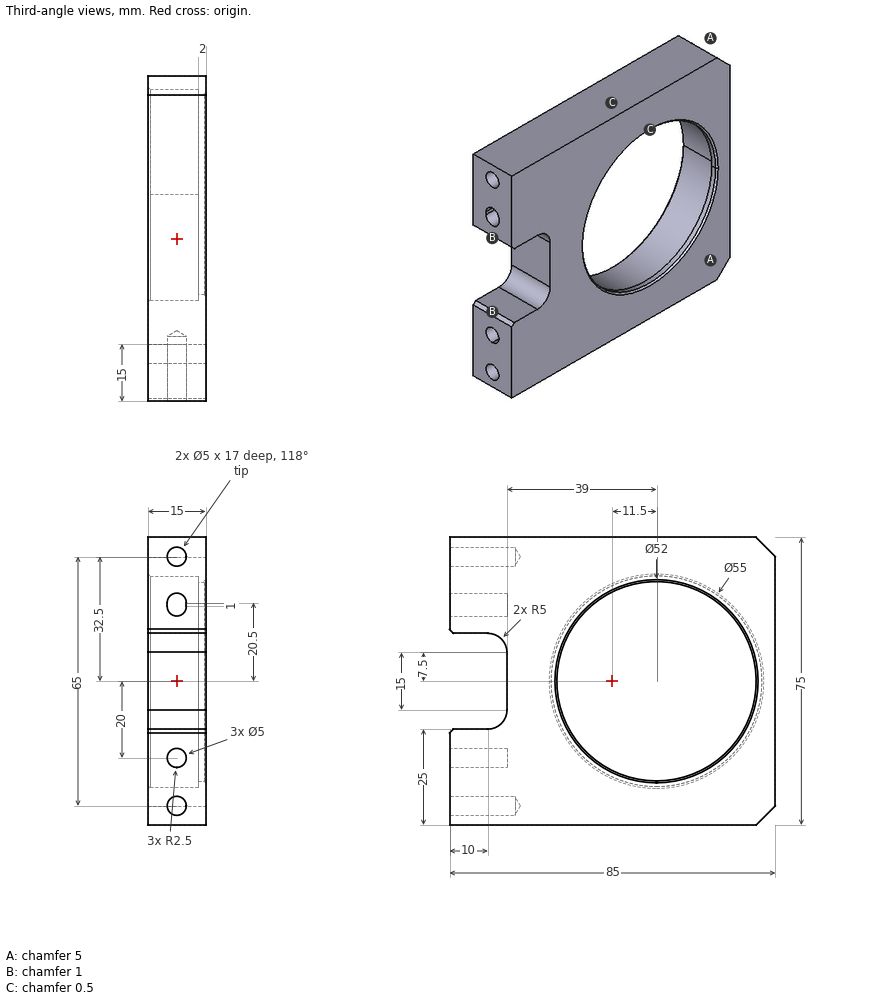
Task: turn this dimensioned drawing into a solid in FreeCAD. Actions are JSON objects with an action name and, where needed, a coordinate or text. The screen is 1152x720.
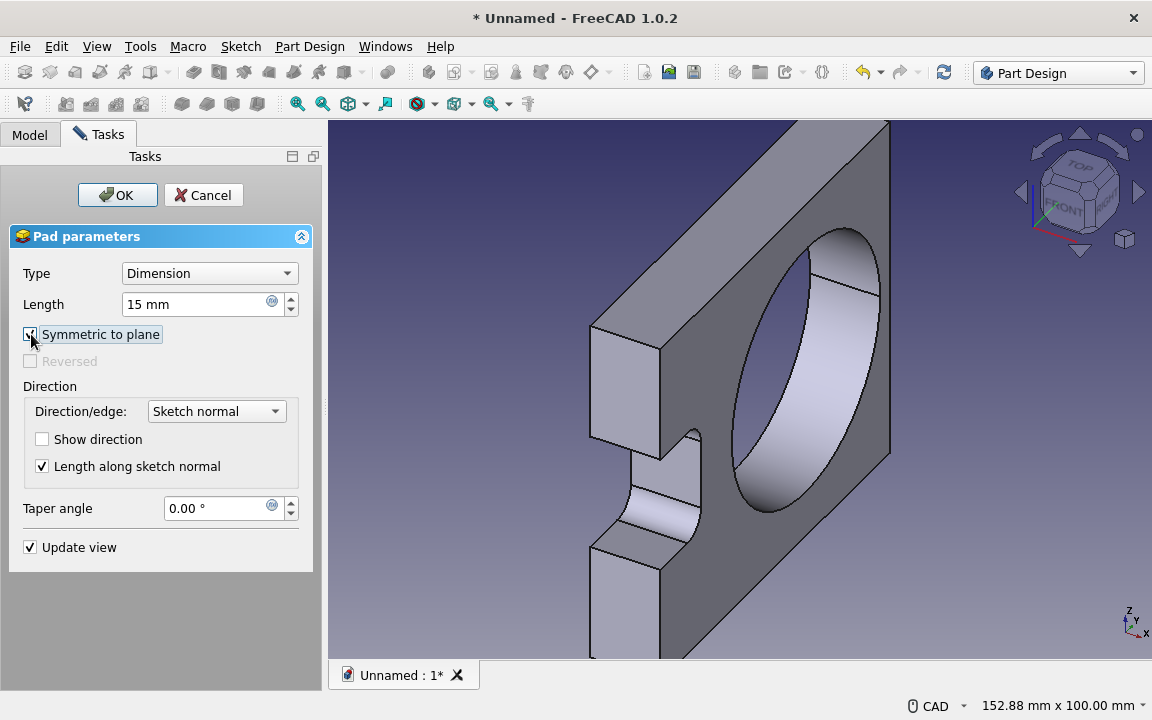
{"action": "left_click", "coordinate": [118, 195]}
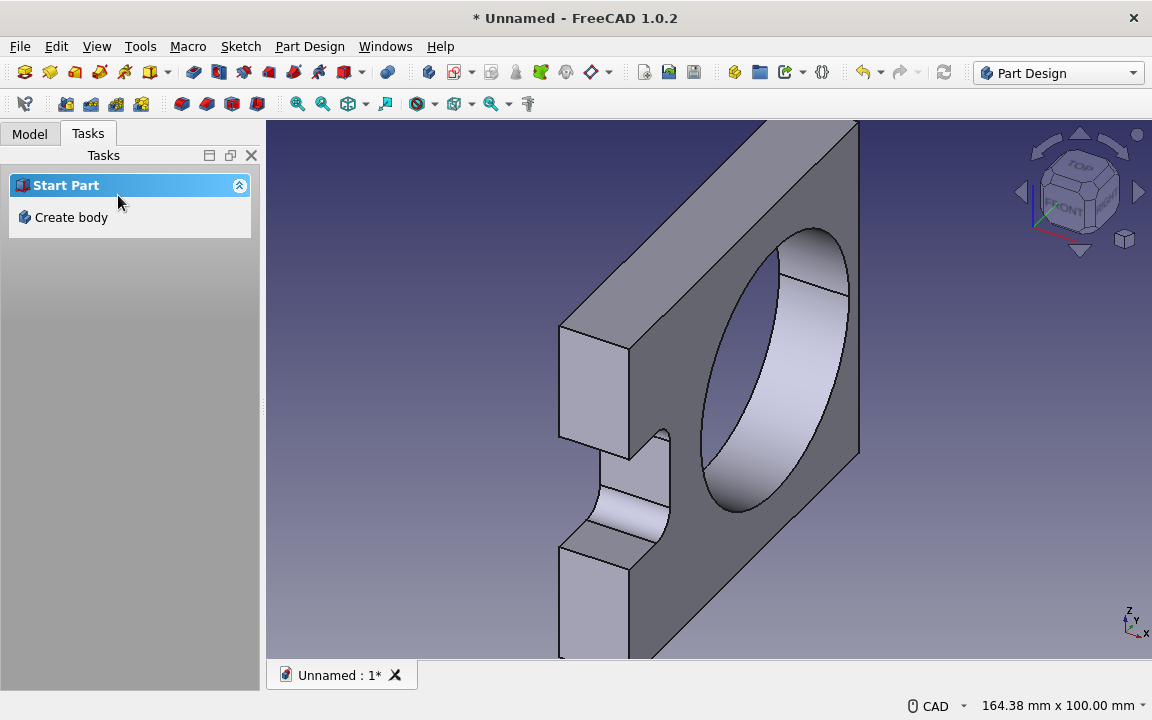
{"action": "left_click", "coordinate": [298, 104]}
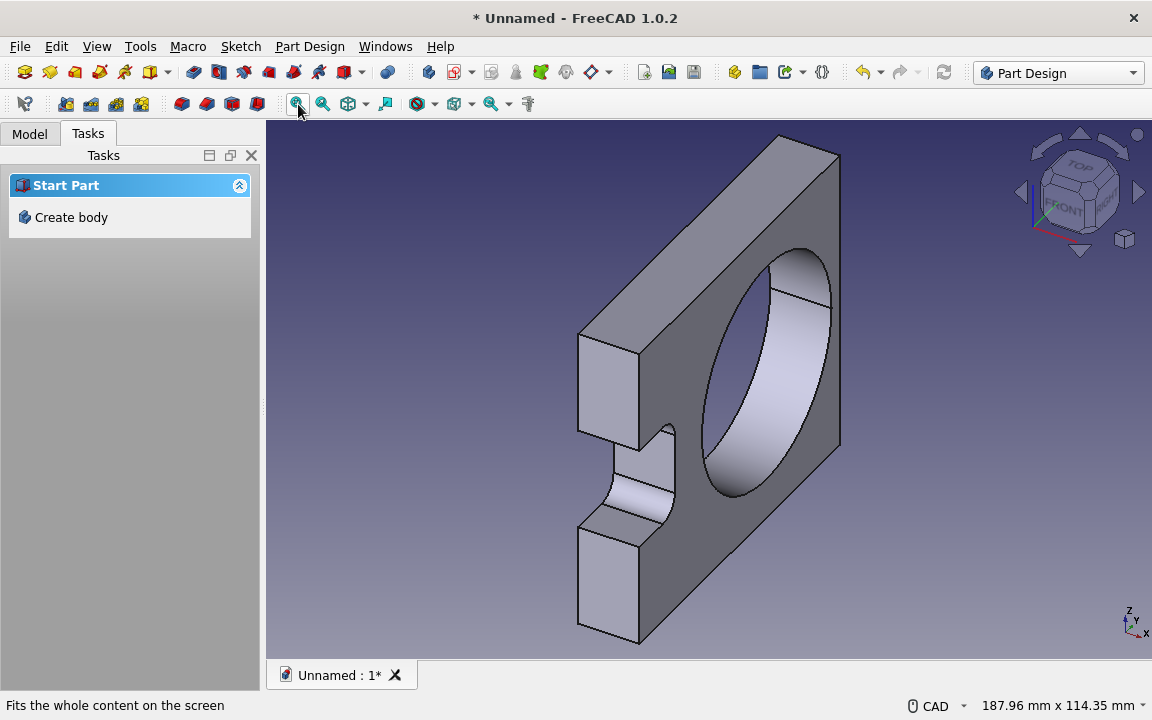
{"action": "left_click", "coordinate": [609, 598]}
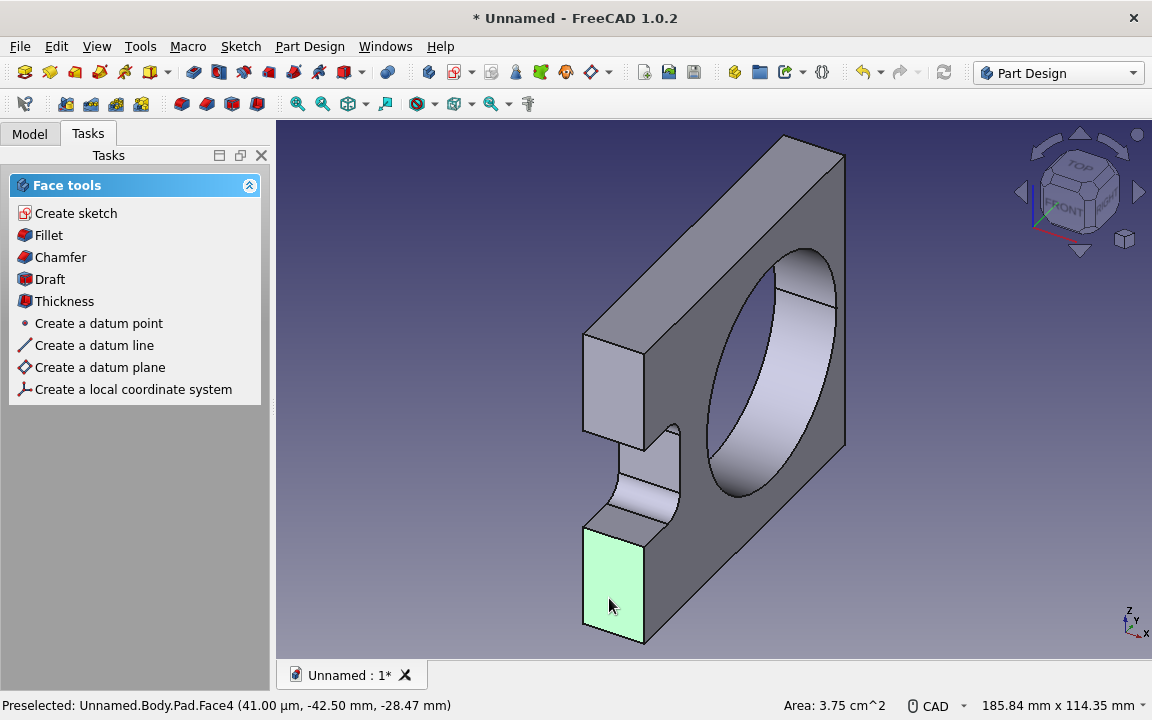
{"action": "left_click", "coordinate": [454, 72]}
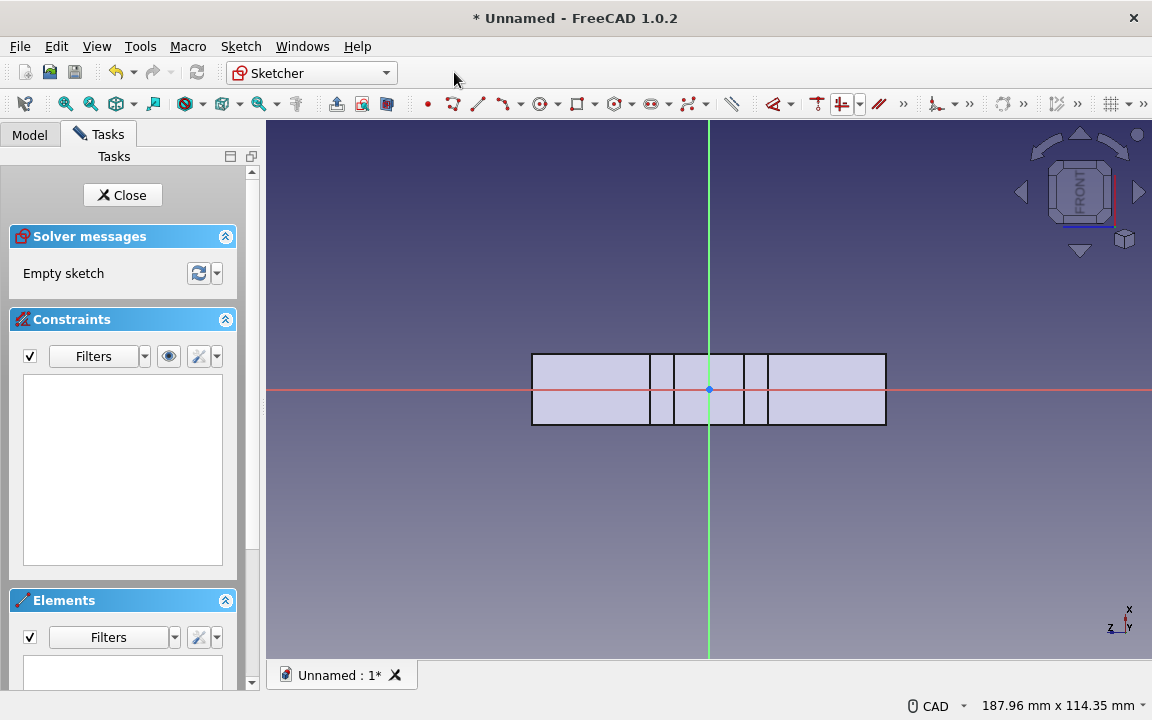
{"action": "scroll", "coordinate": [848, 390], "scroll_direction": "up", "scroll_amount": 2}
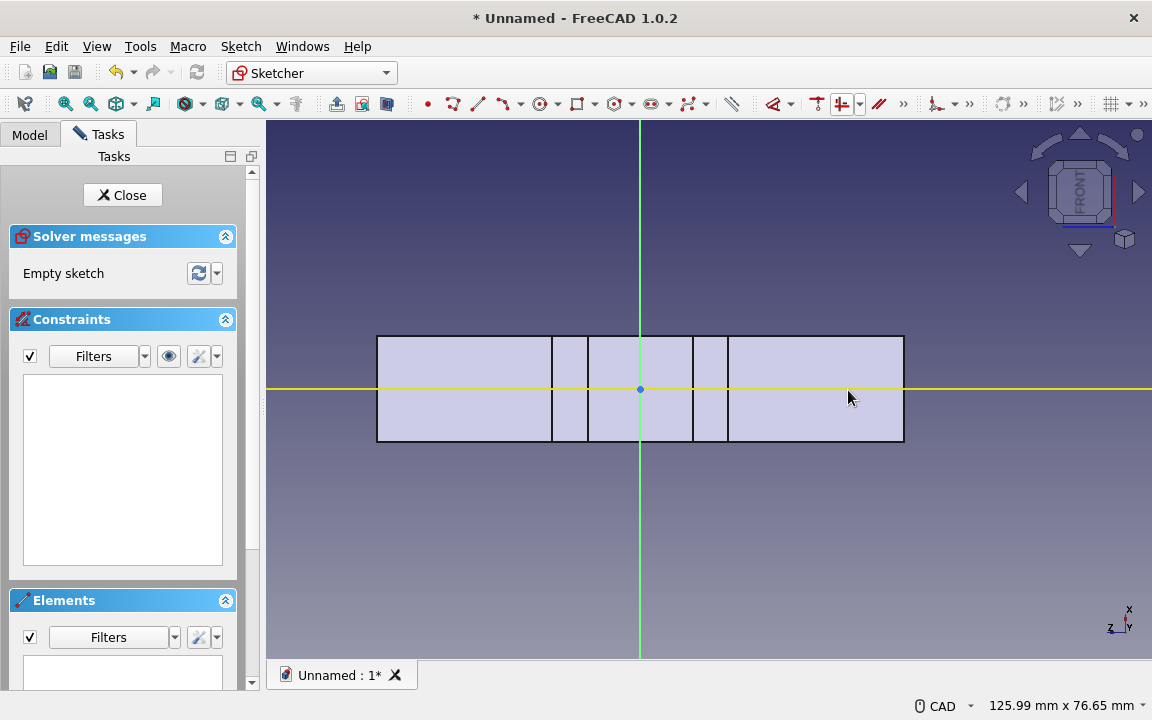
{"action": "left_click", "coordinate": [540, 104]}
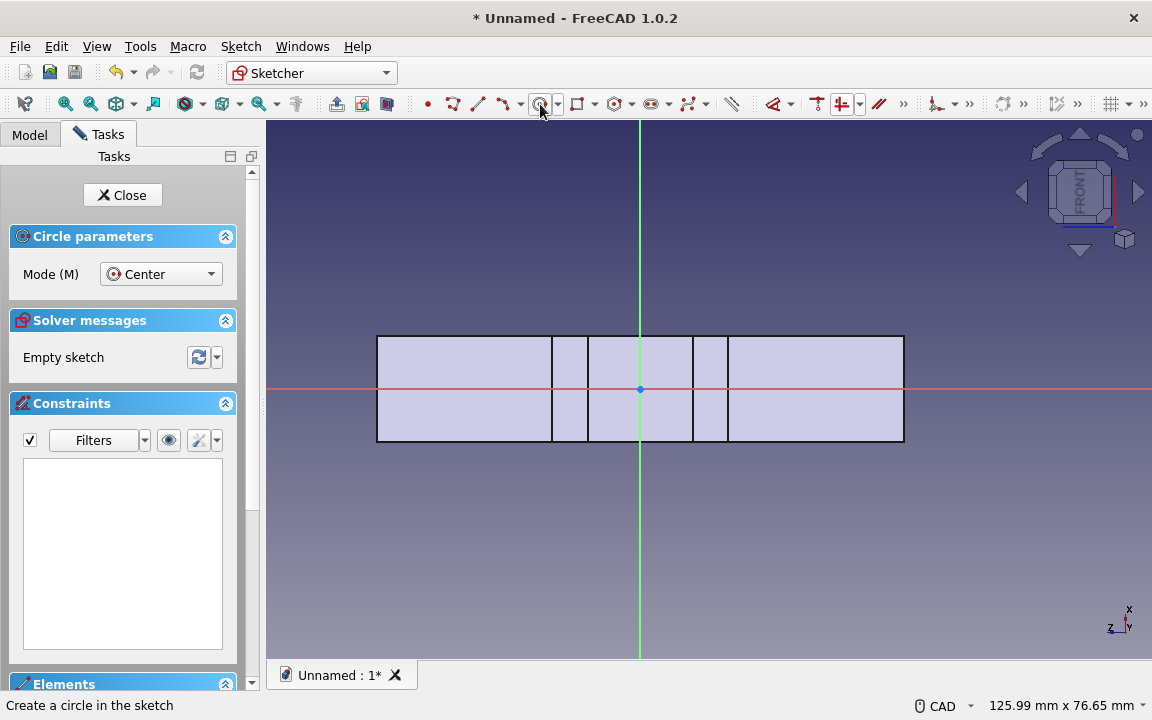
{"action": "scroll", "coordinate": [412, 389], "scroll_direction": "up", "scroll_amount": 2}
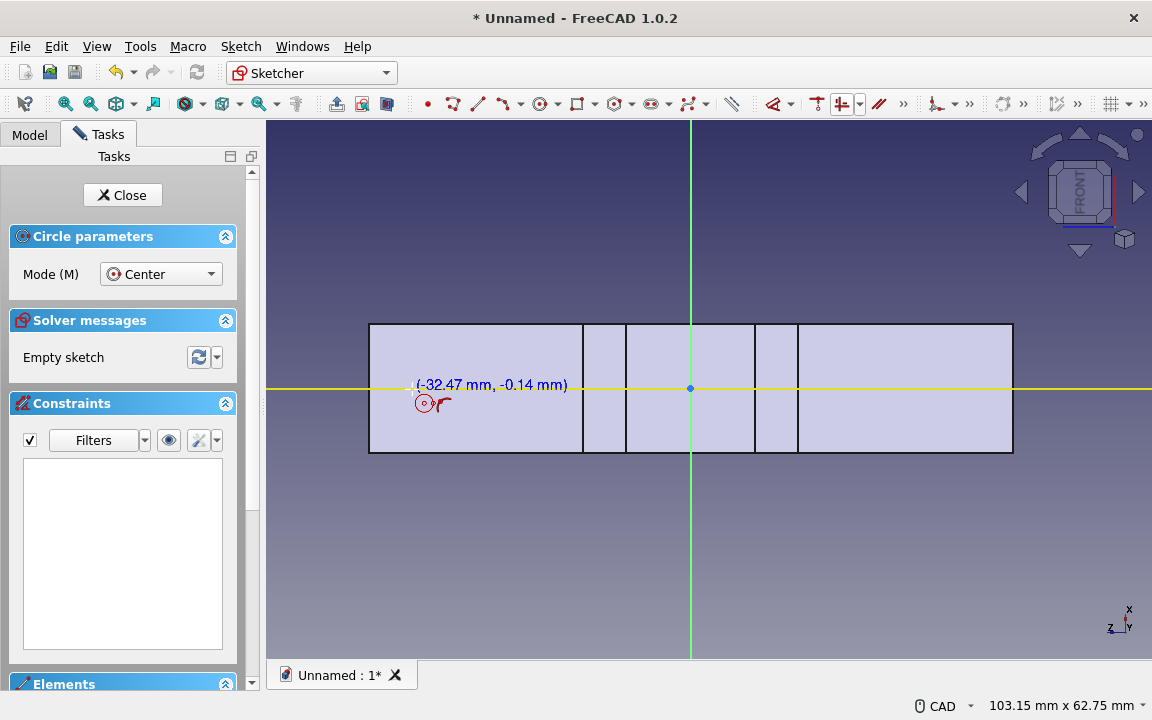
{"action": "left_click", "coordinate": [412, 389]}
{"action": "mouse_move", "coordinate": [430, 370]}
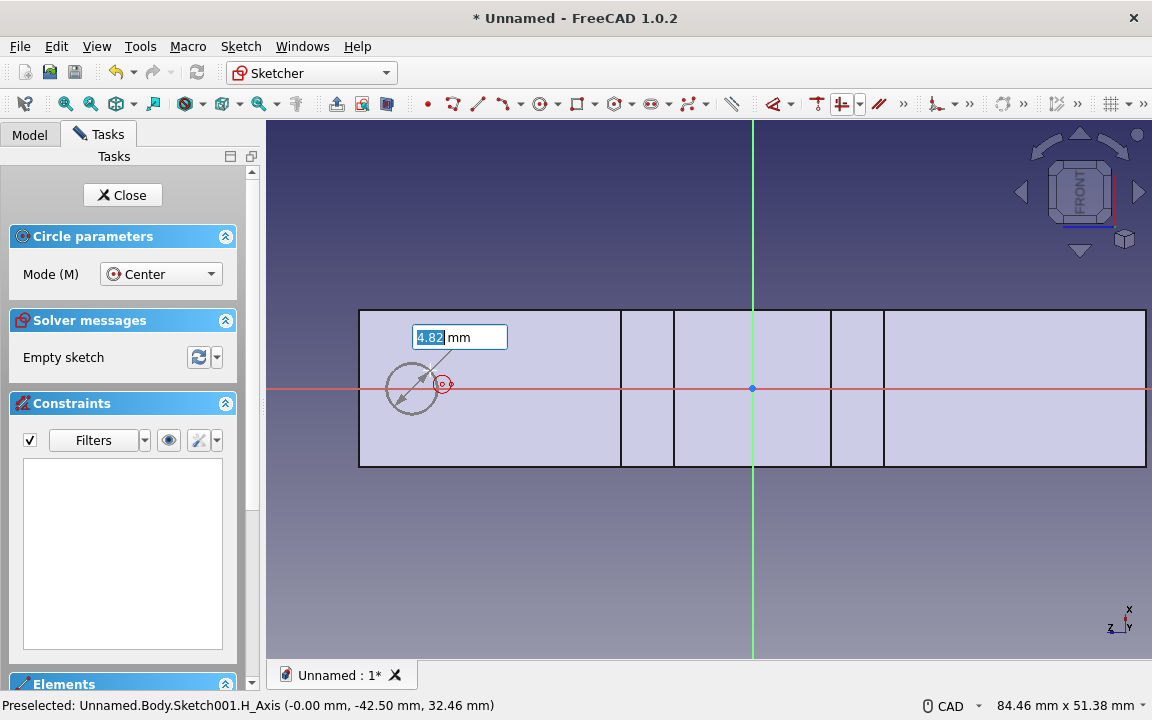
{"action": "type", "text": "5"}
{"action": "key", "text": "Return"}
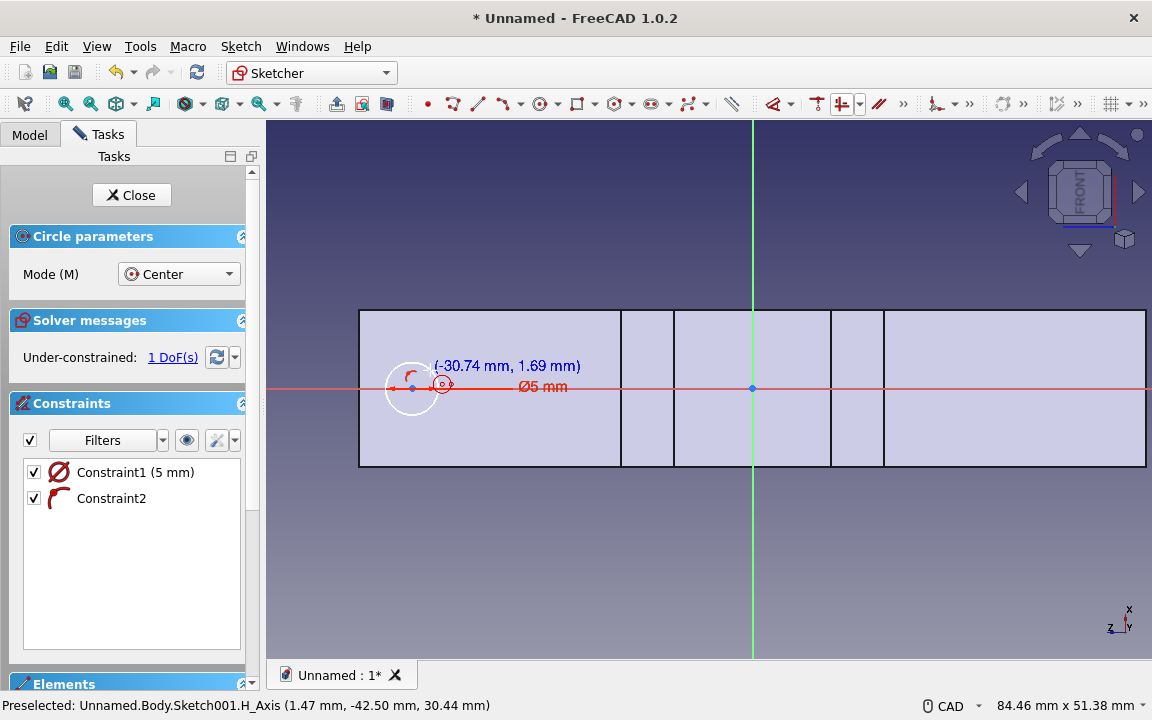
{"action": "scroll", "coordinate": [413, 391], "scroll_direction": "down", "scroll_amount": 2}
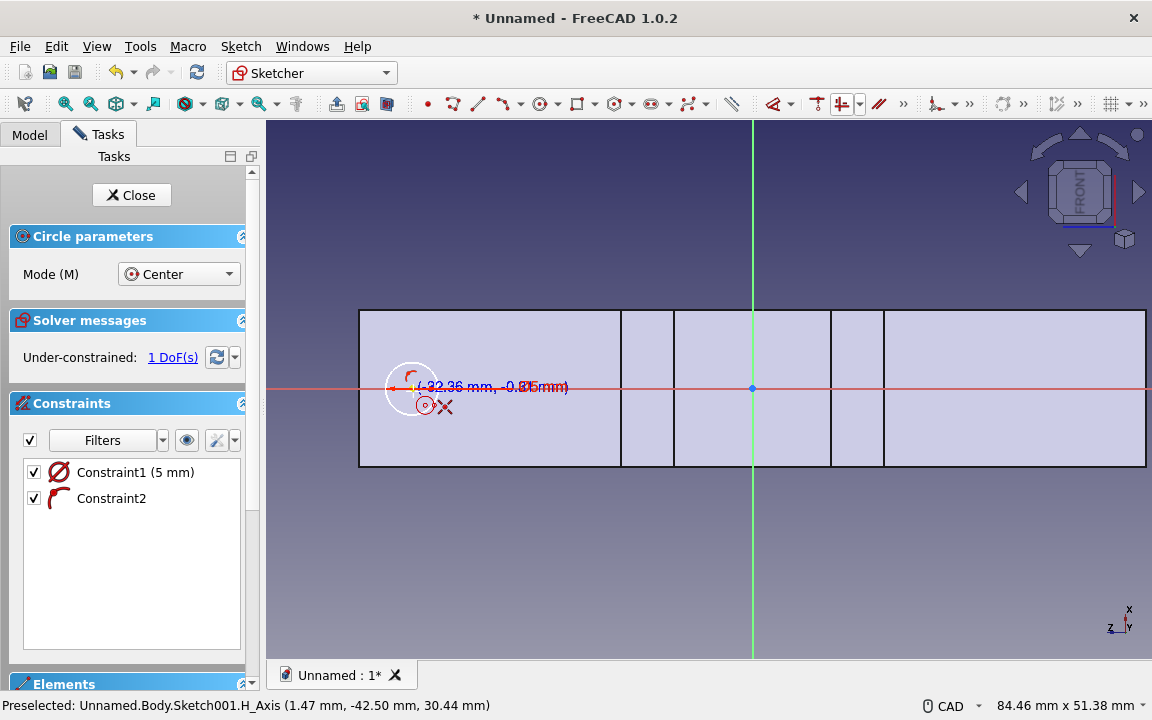
{"action": "scroll", "coordinate": [869, 390], "scroll_direction": "up", "scroll_amount": 2}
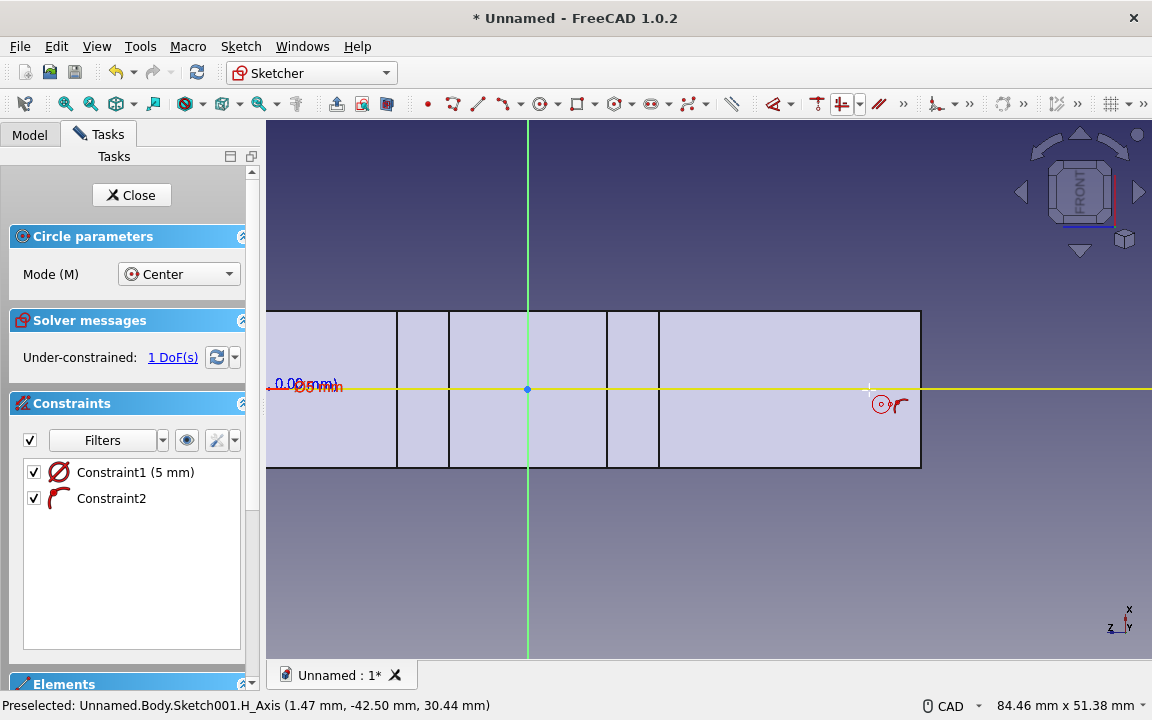
{"action": "left_click", "coordinate": [869, 389]}
{"action": "mouse_move", "coordinate": [887, 371]}